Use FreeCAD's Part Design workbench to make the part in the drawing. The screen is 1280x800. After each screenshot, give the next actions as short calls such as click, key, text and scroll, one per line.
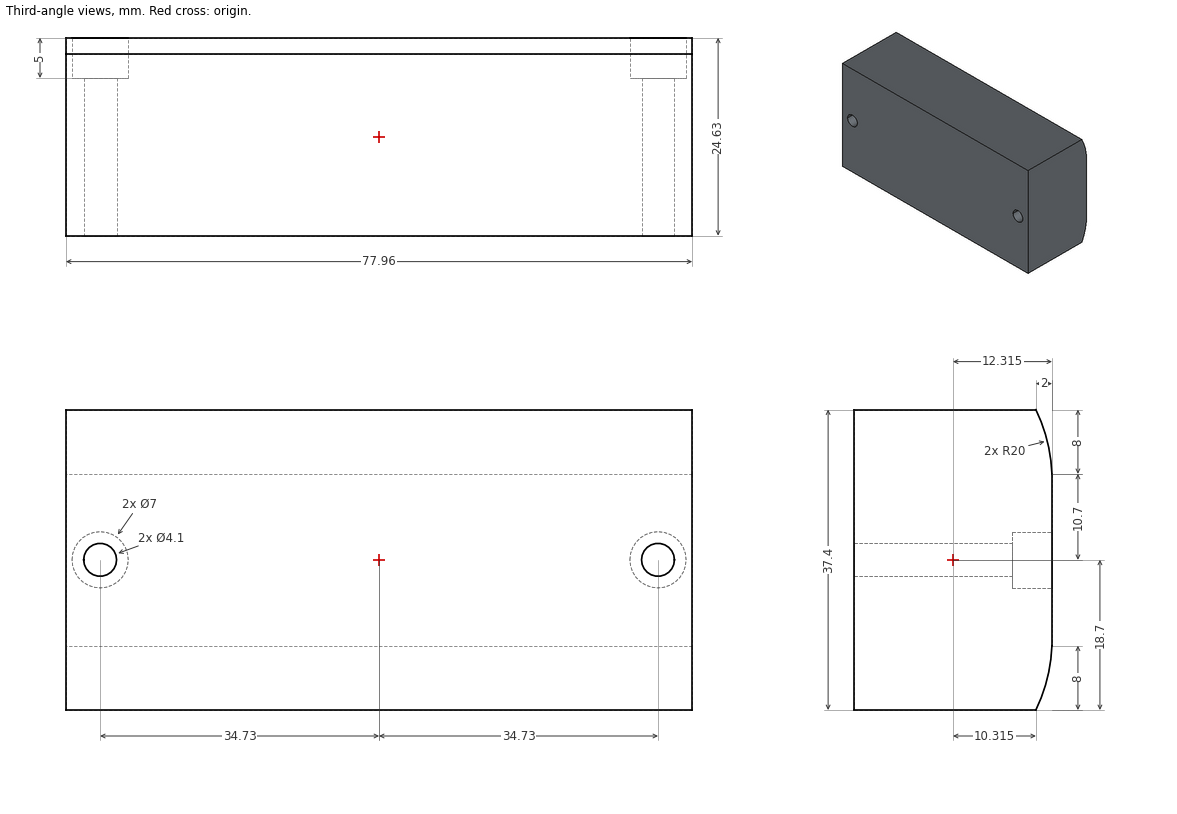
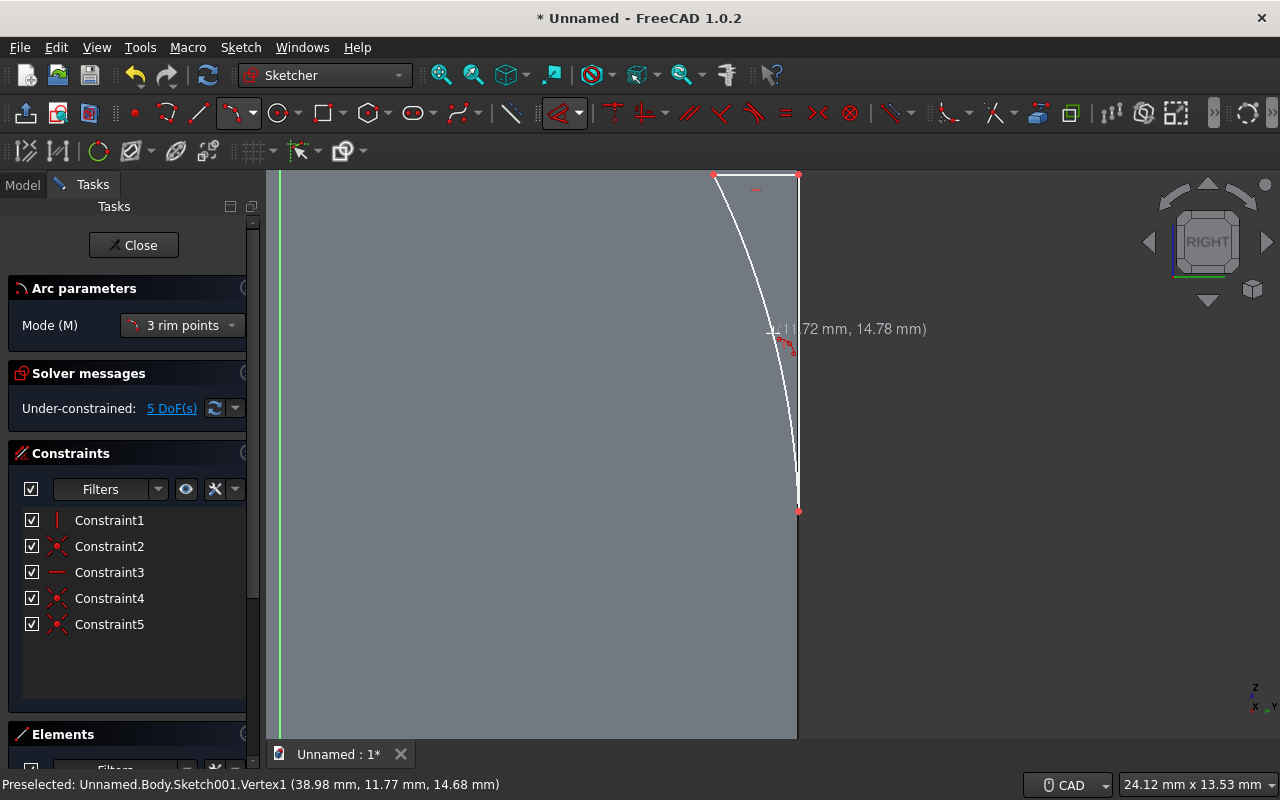
click(168, 114)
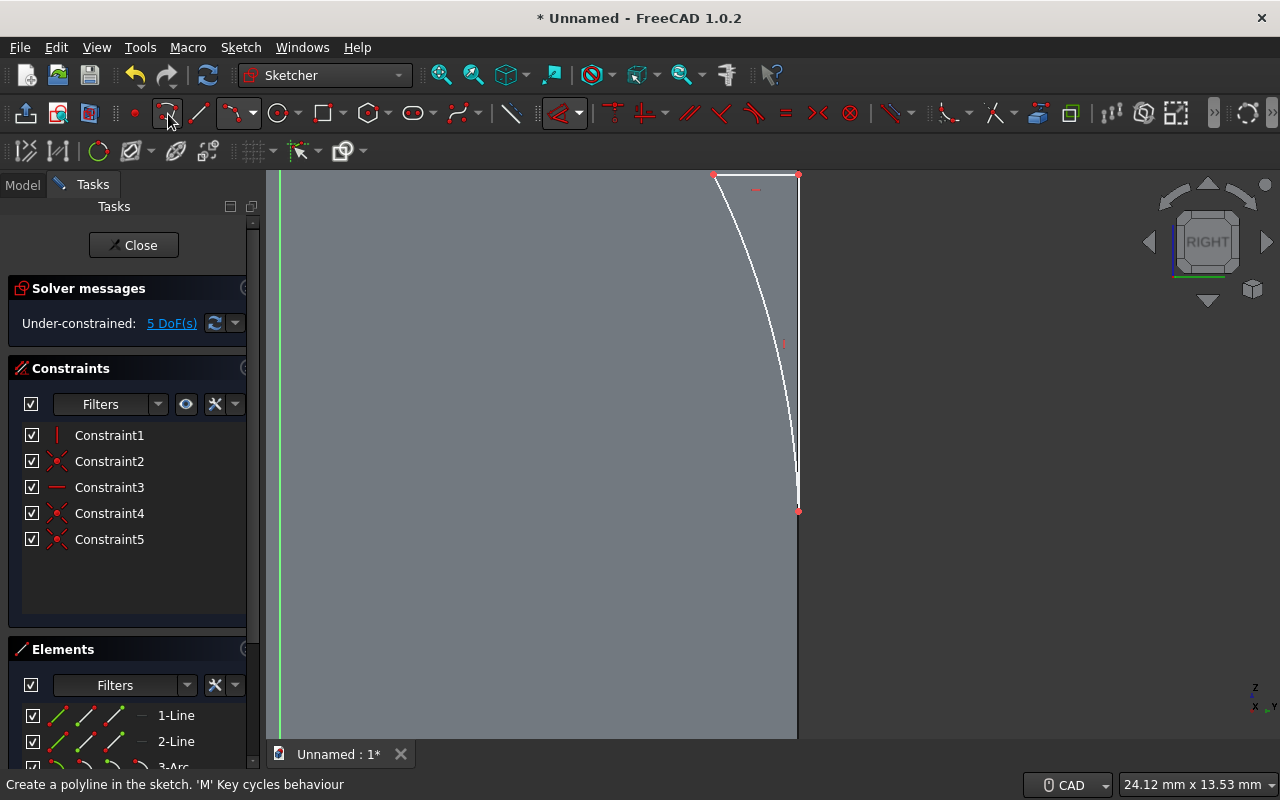
scroll(759, 290, down, 7)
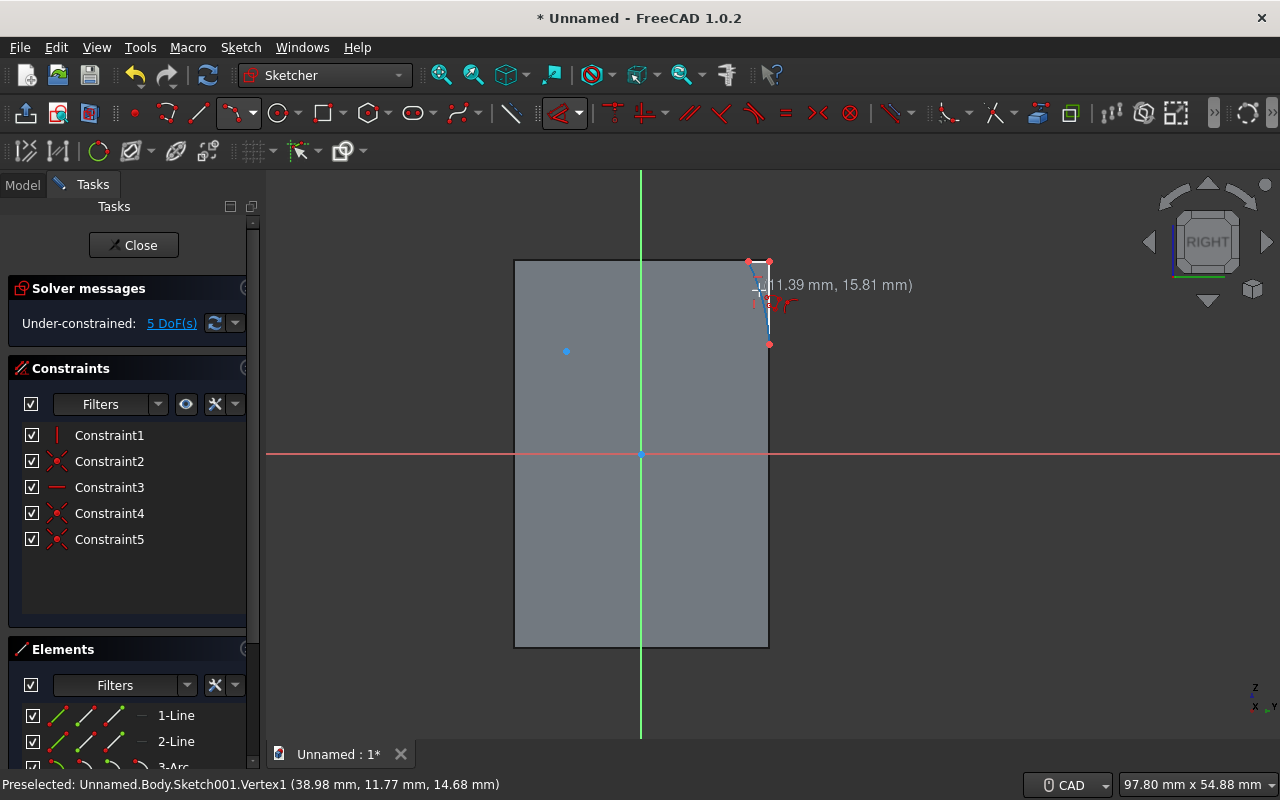
click(748, 648)
click(769, 648)
click(769, 565)
right_click(769, 565)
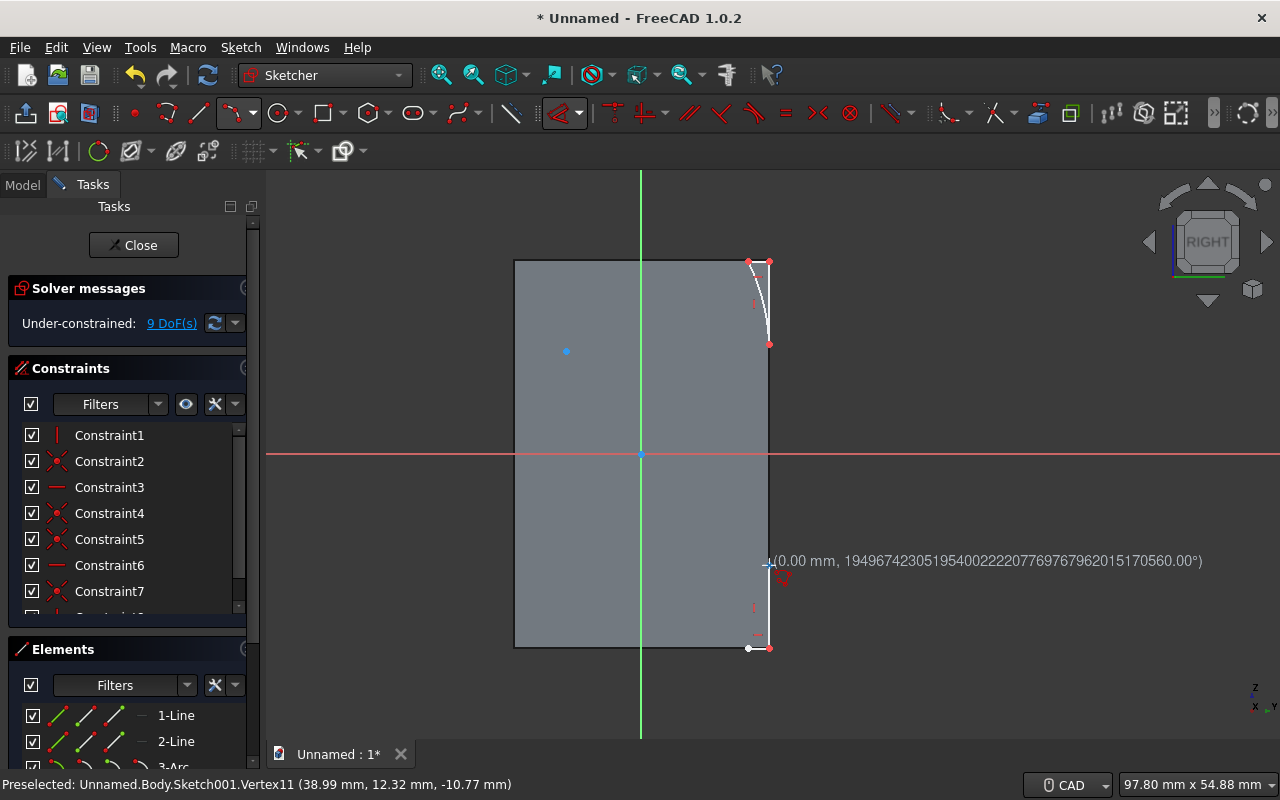
click(232, 114)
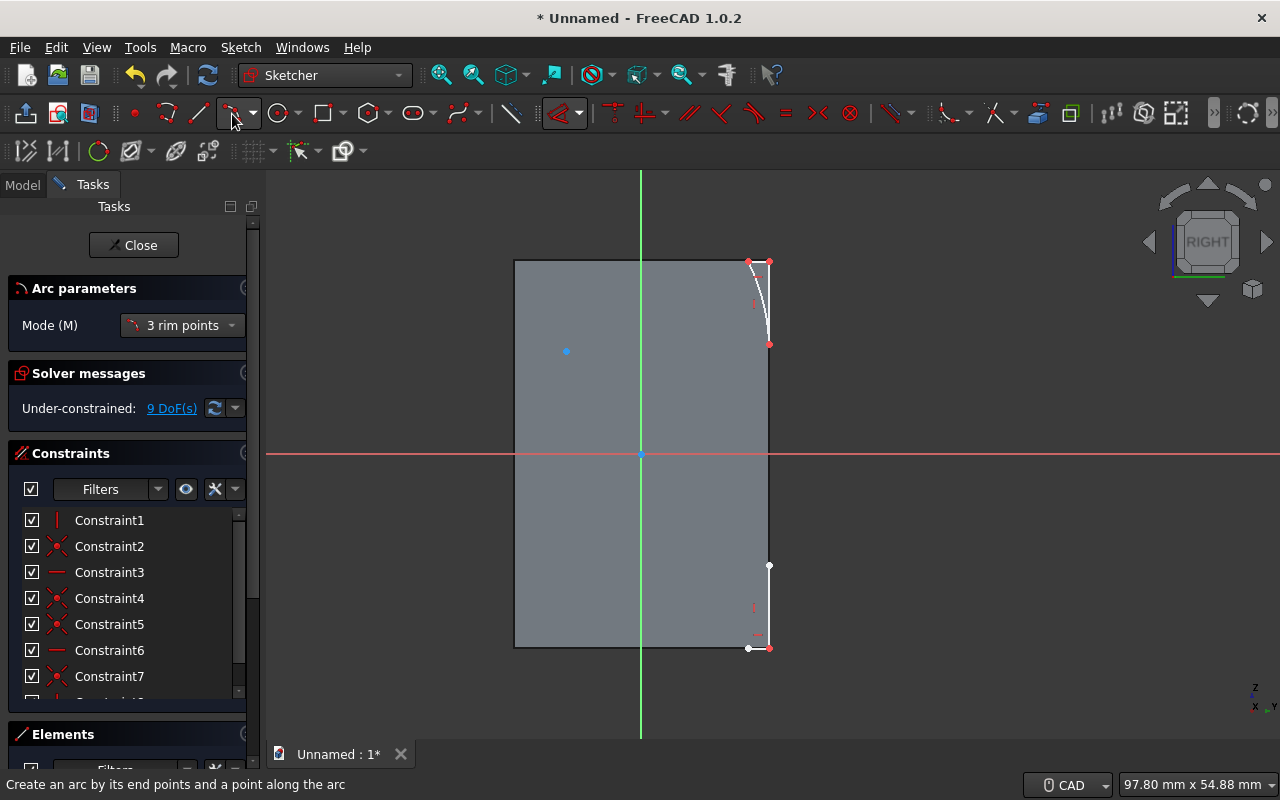
click(769, 566)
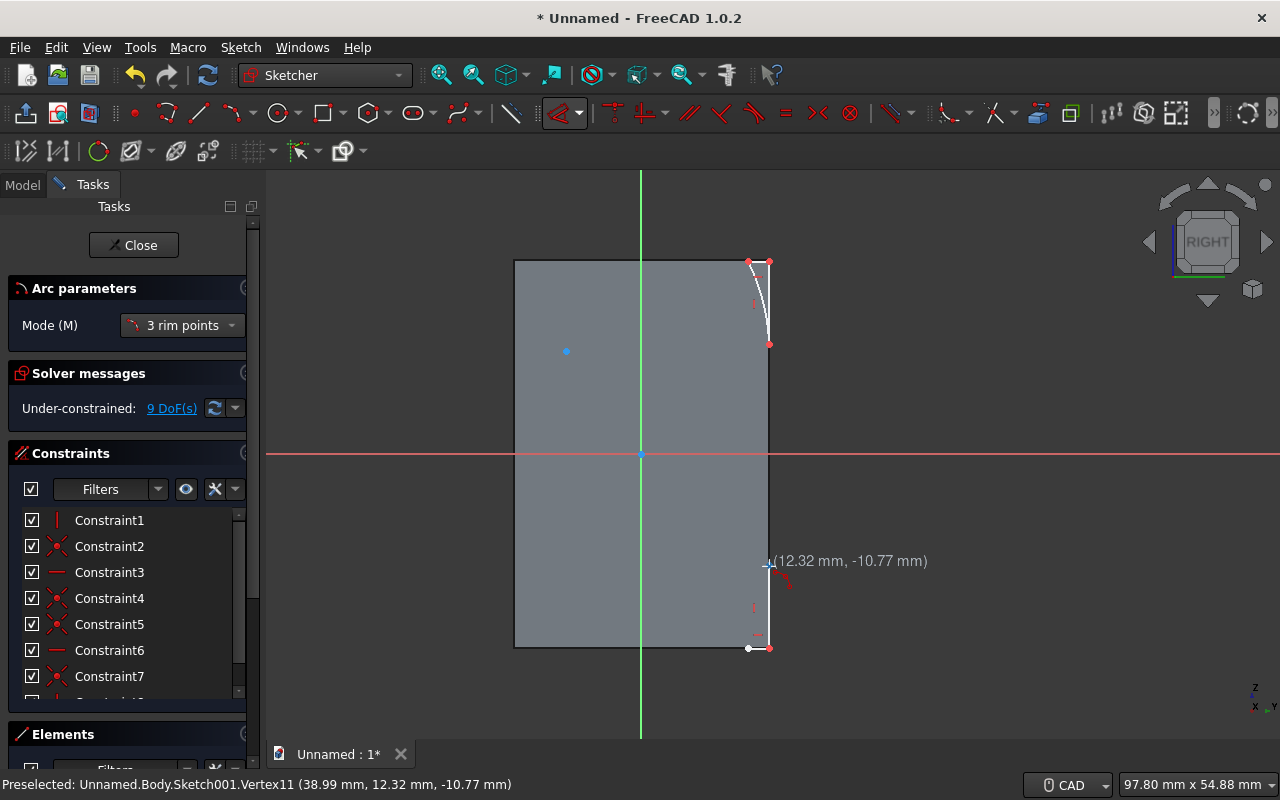
scroll(748, 648, up, 3)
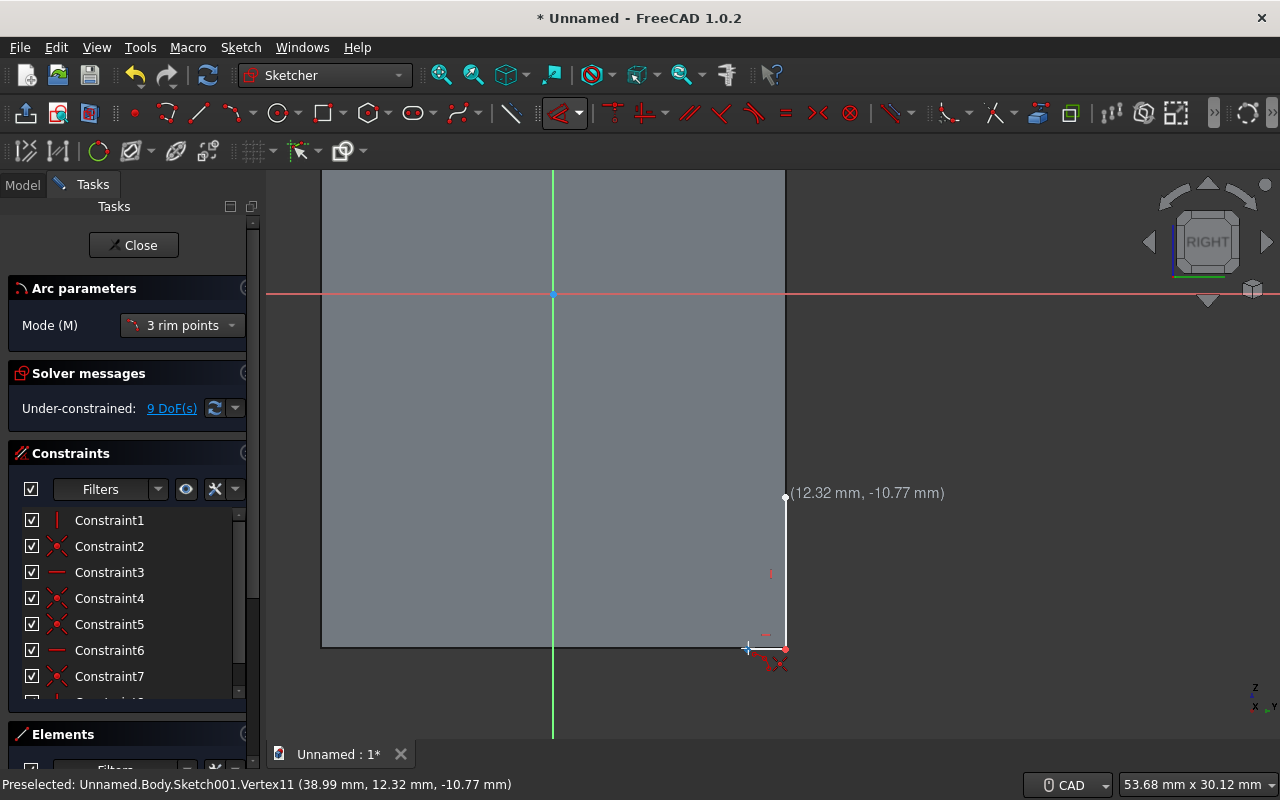
click(748, 649)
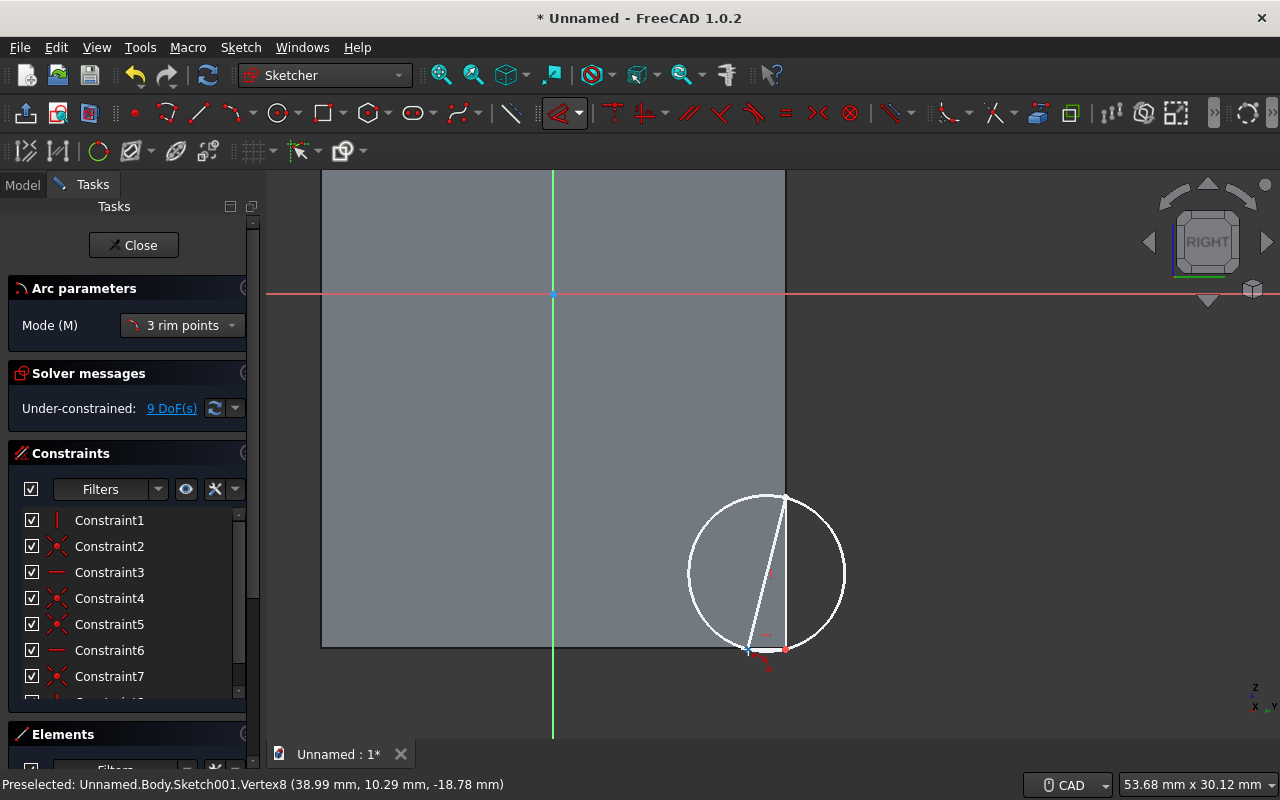
scroll(775, 574, up, 4)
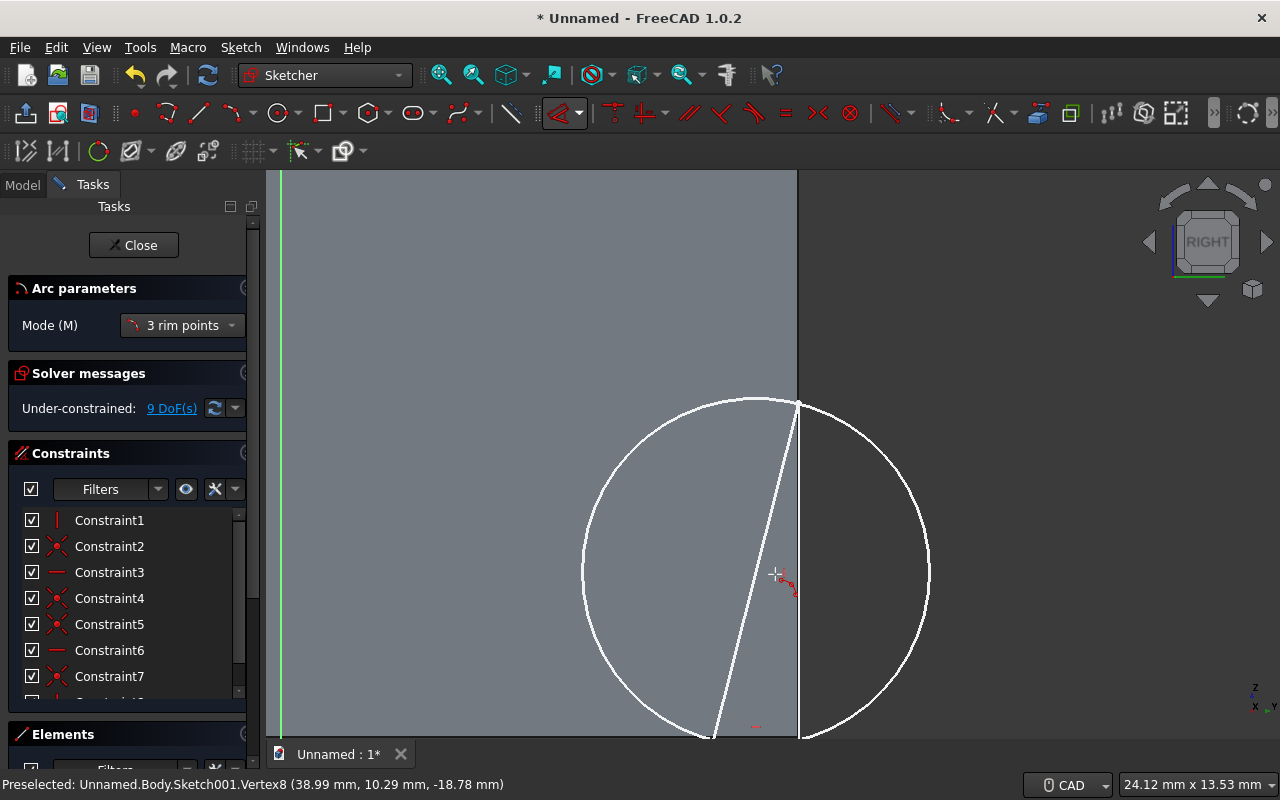
click(774, 573)
key(Escape)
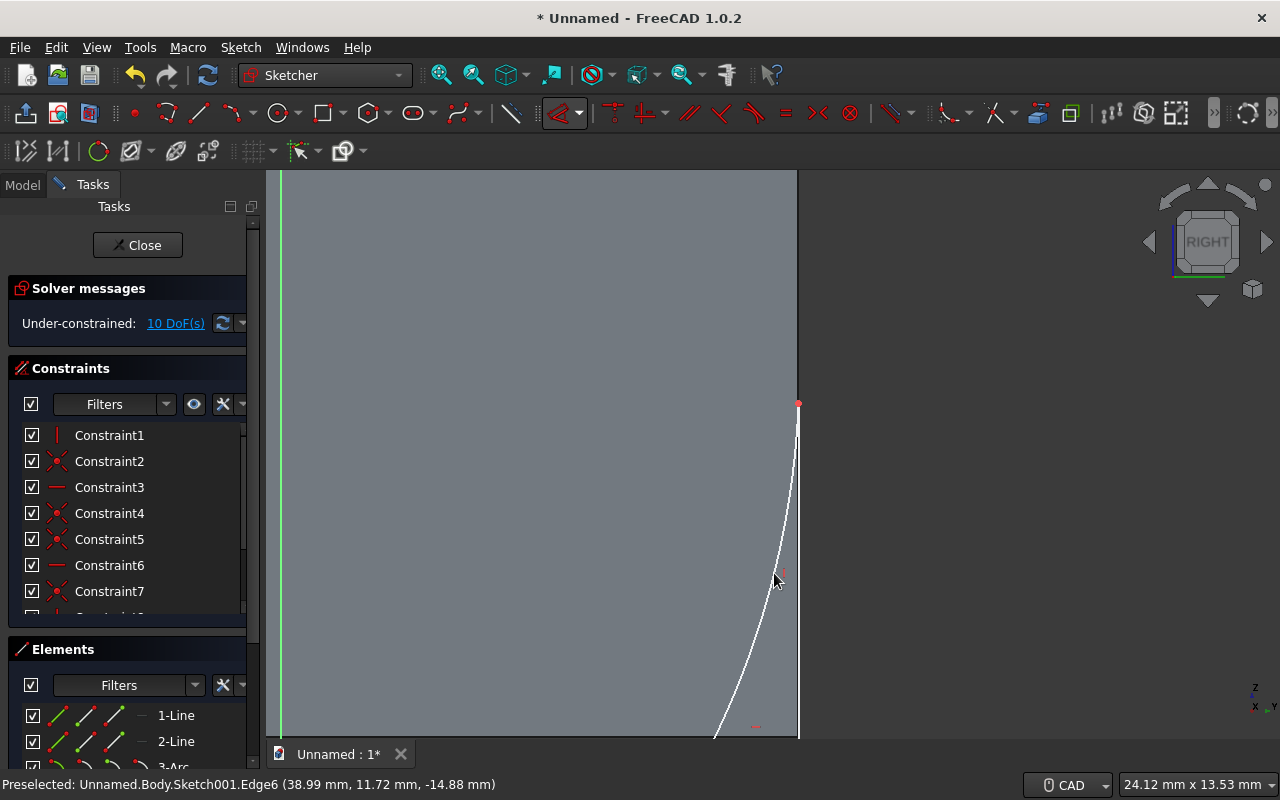
scroll(758, 619, down, 7)